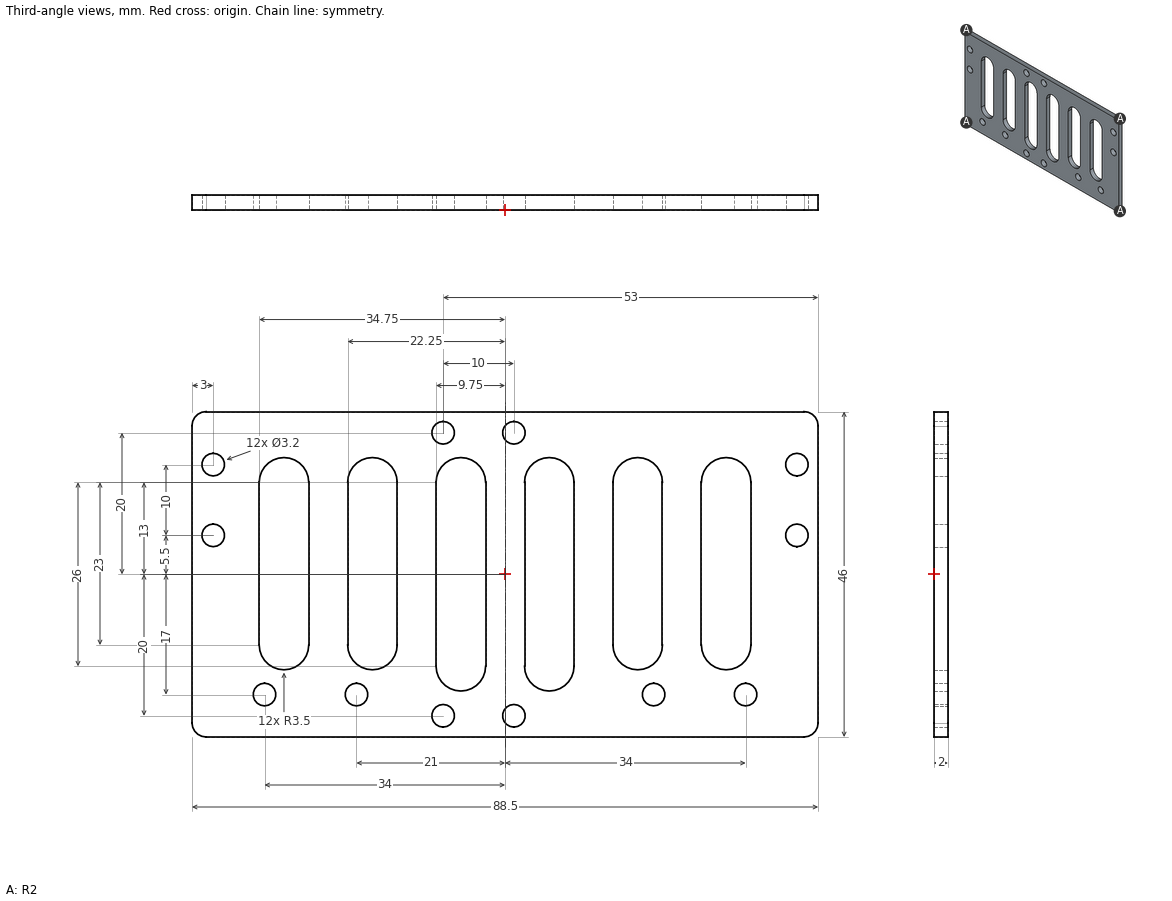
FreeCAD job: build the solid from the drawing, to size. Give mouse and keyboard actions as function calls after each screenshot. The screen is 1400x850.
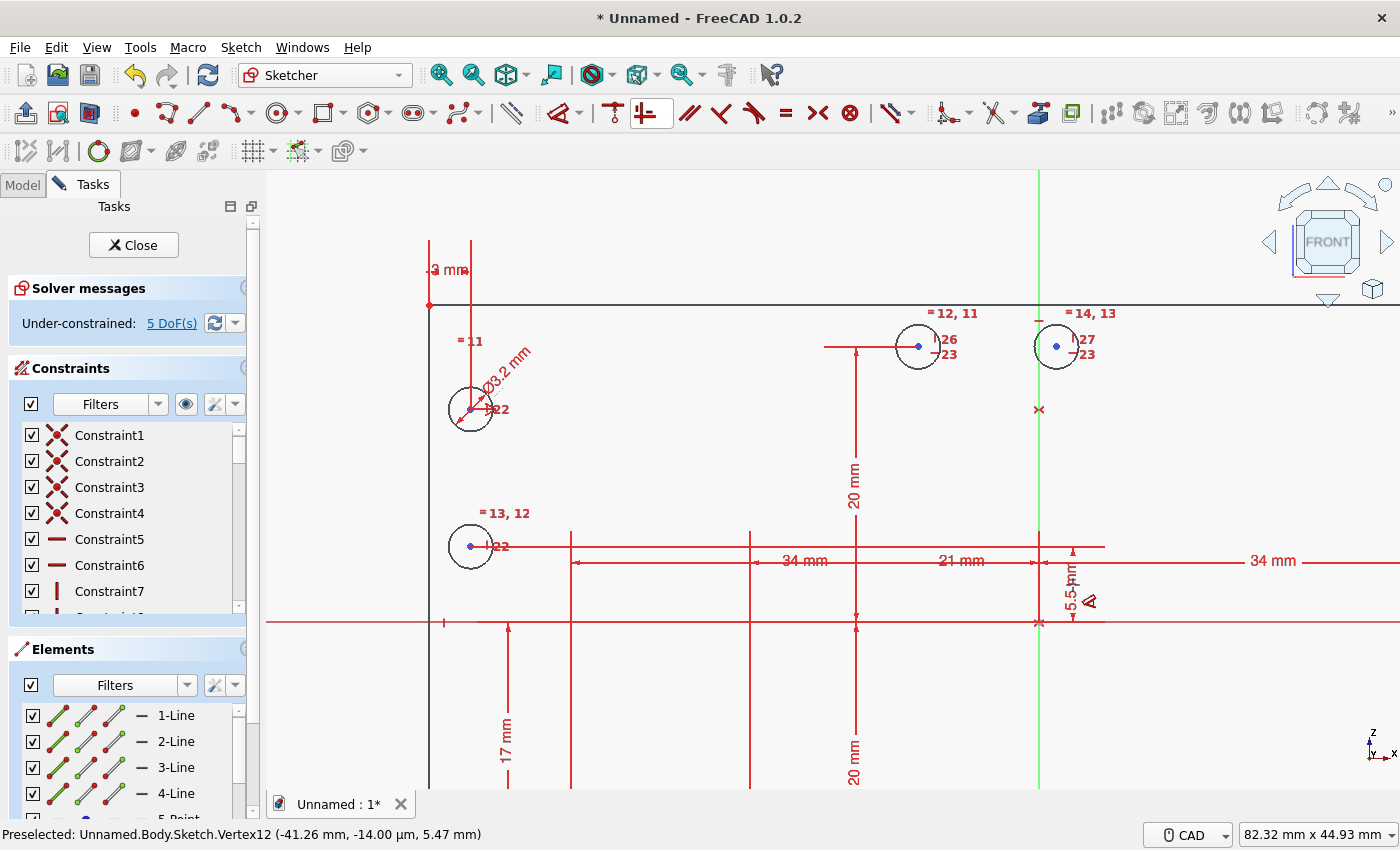
scroll(430, 306, down, 3)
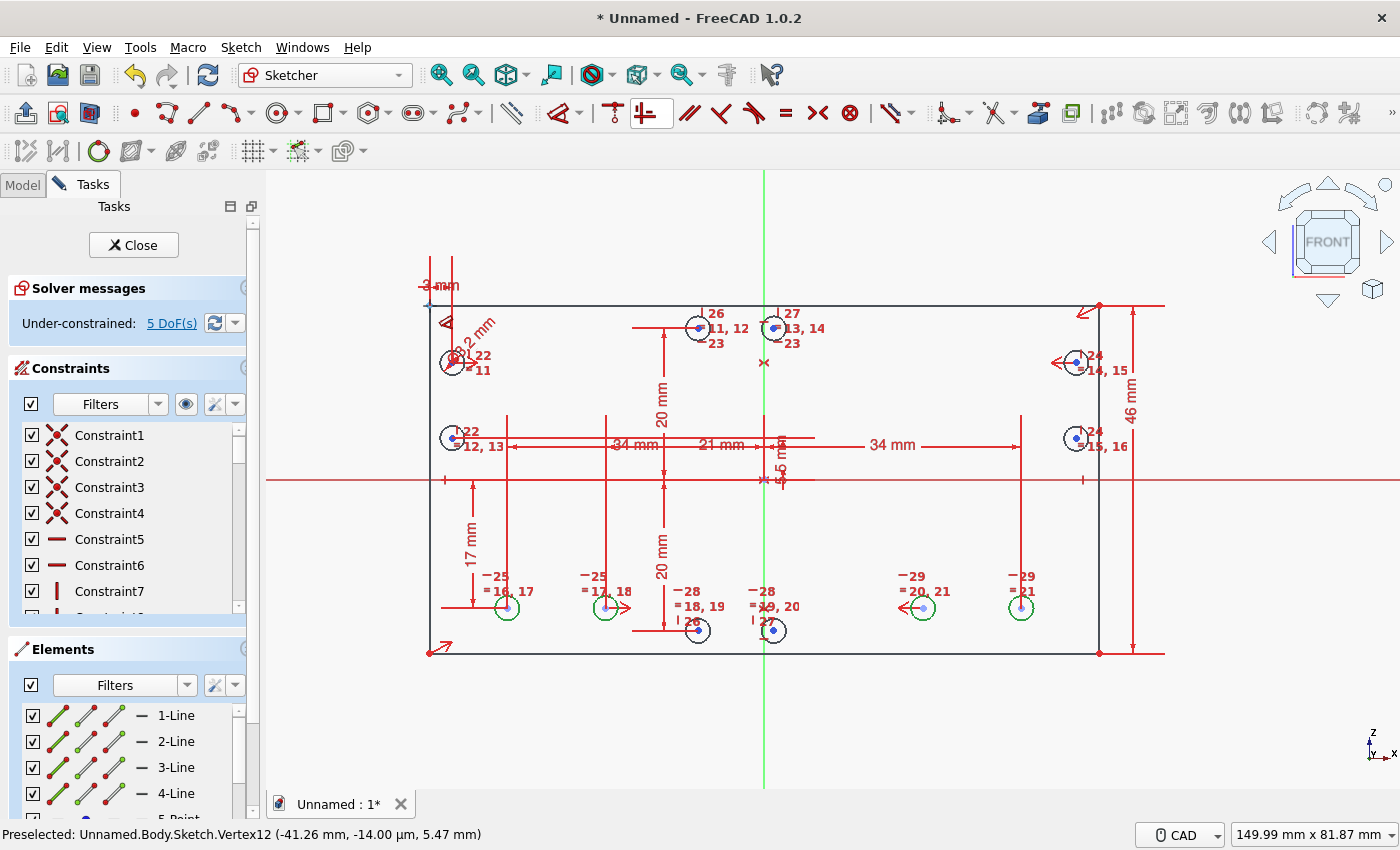
click(1076, 439)
click(1134, 459)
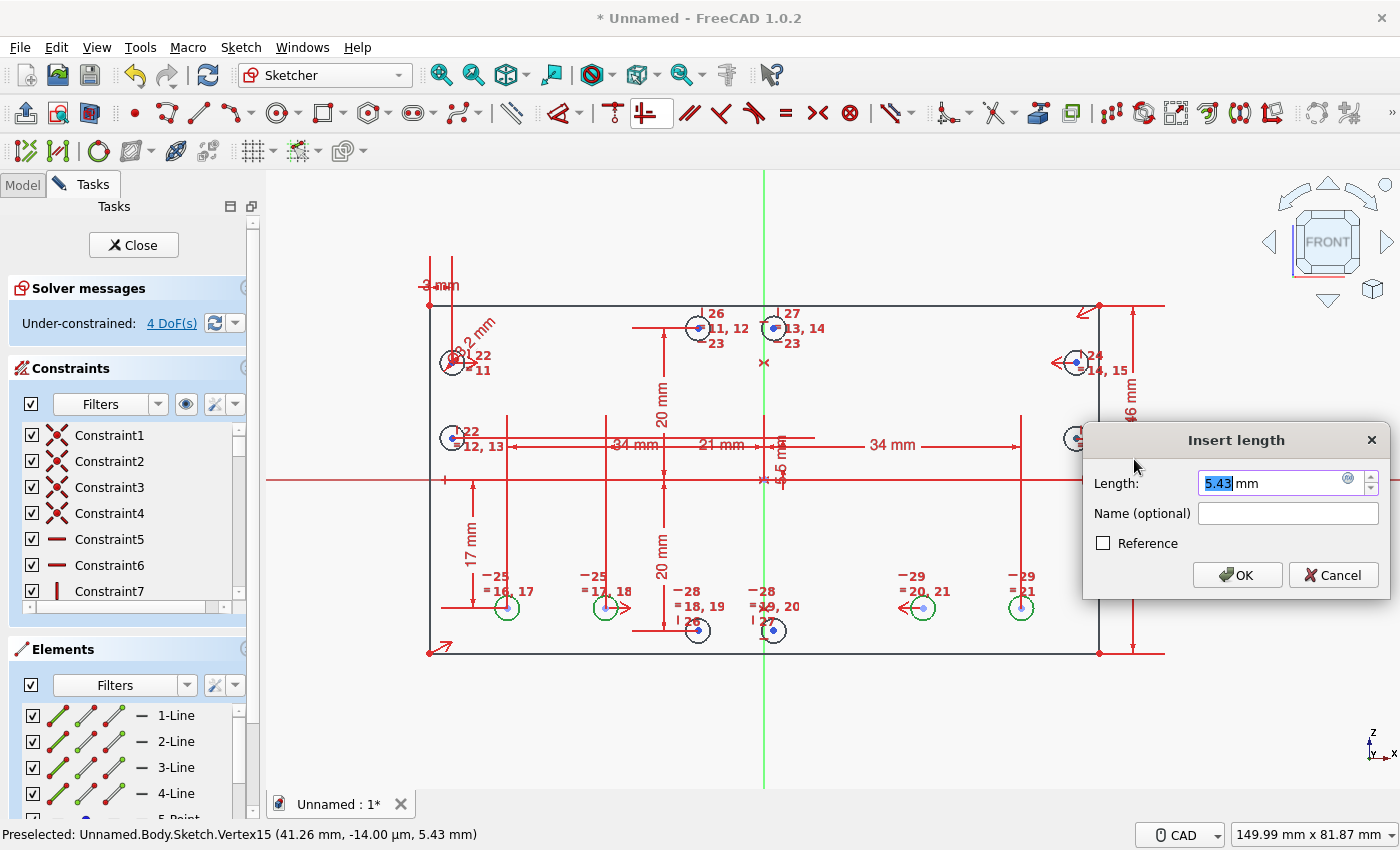
text(5.5)
key(Return)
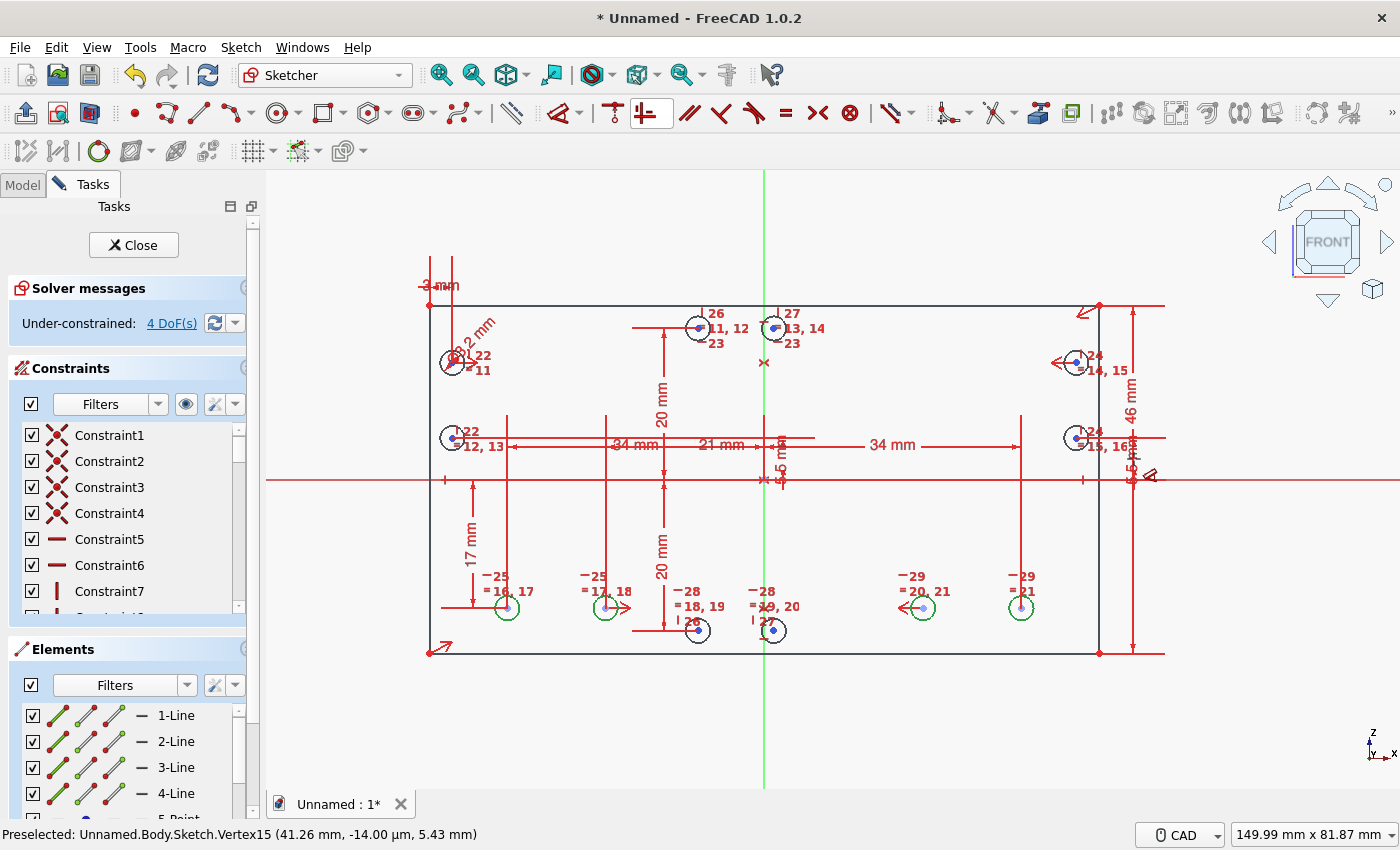
click(1099, 306)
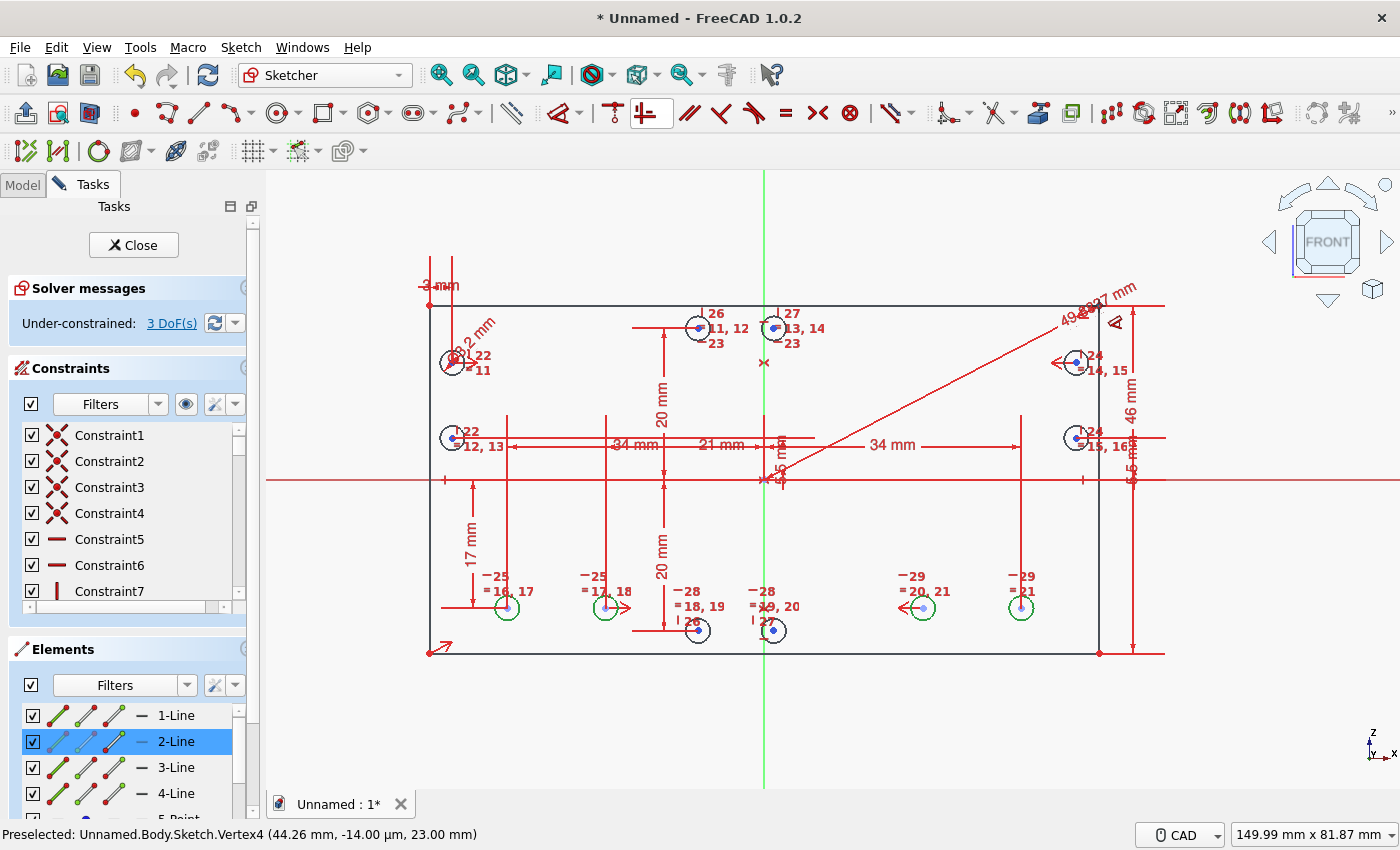
click(698, 328)
click(899, 272)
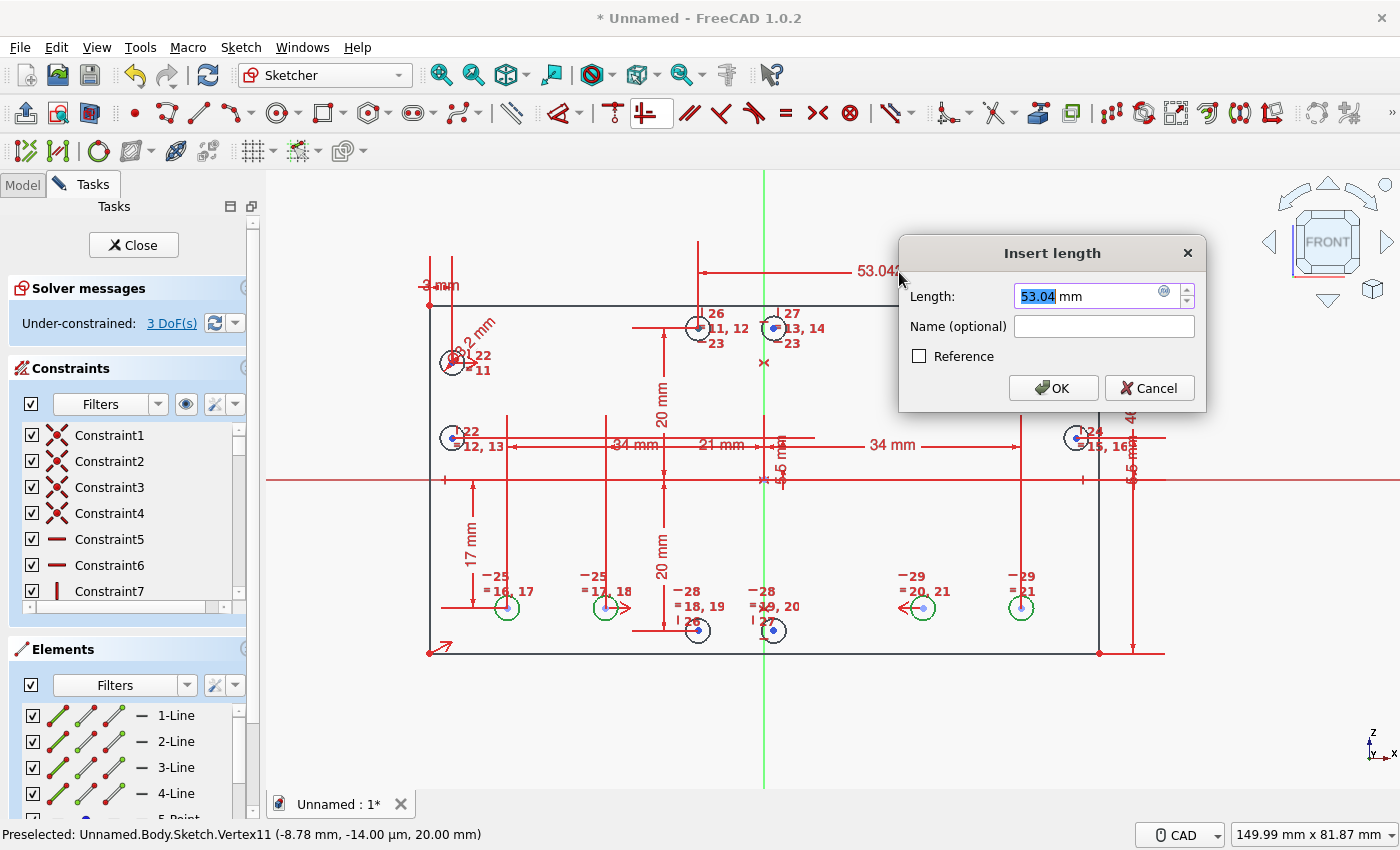
text(53)
key(Return)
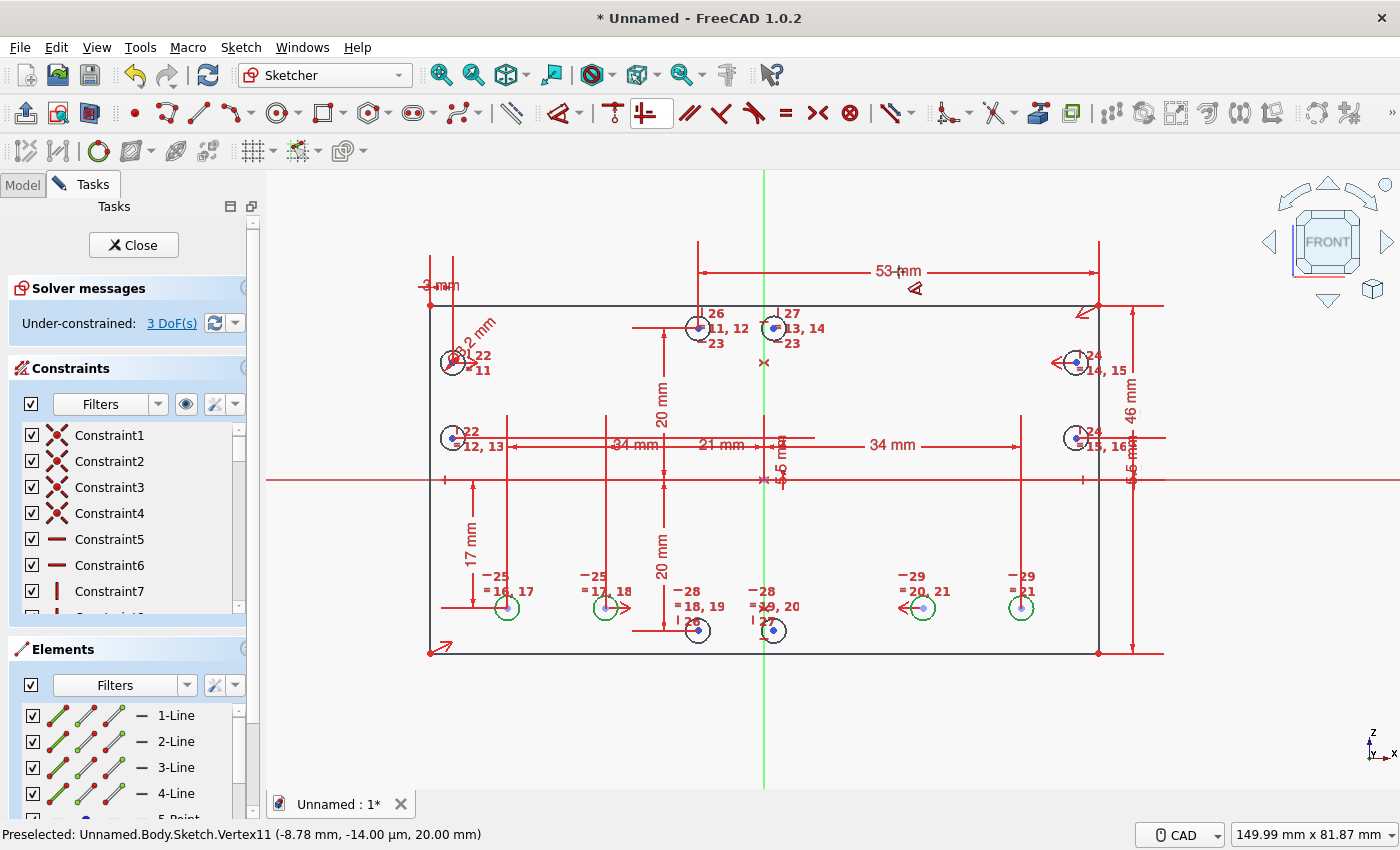
click(453, 363)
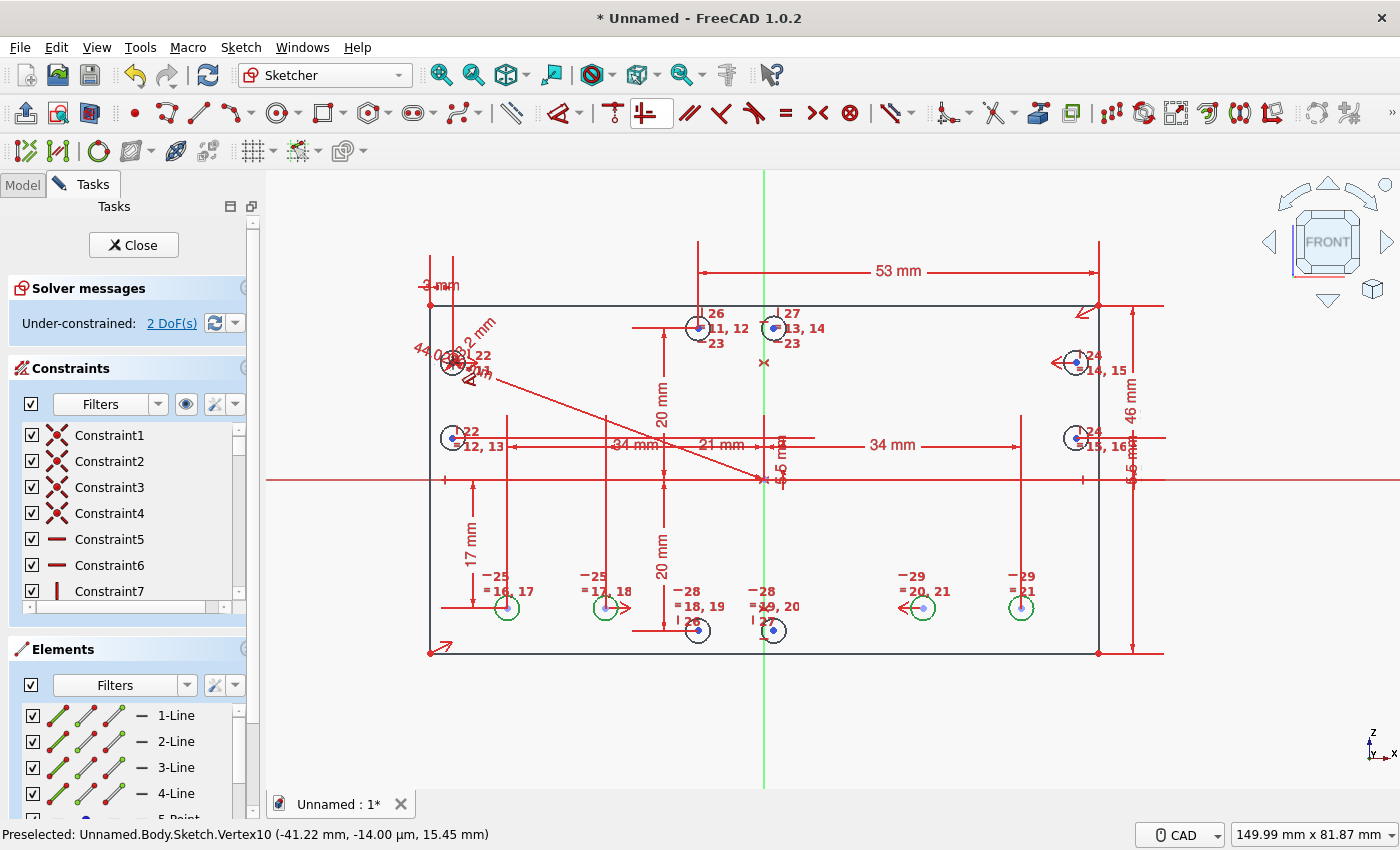
click(453, 438)
click(487, 401)